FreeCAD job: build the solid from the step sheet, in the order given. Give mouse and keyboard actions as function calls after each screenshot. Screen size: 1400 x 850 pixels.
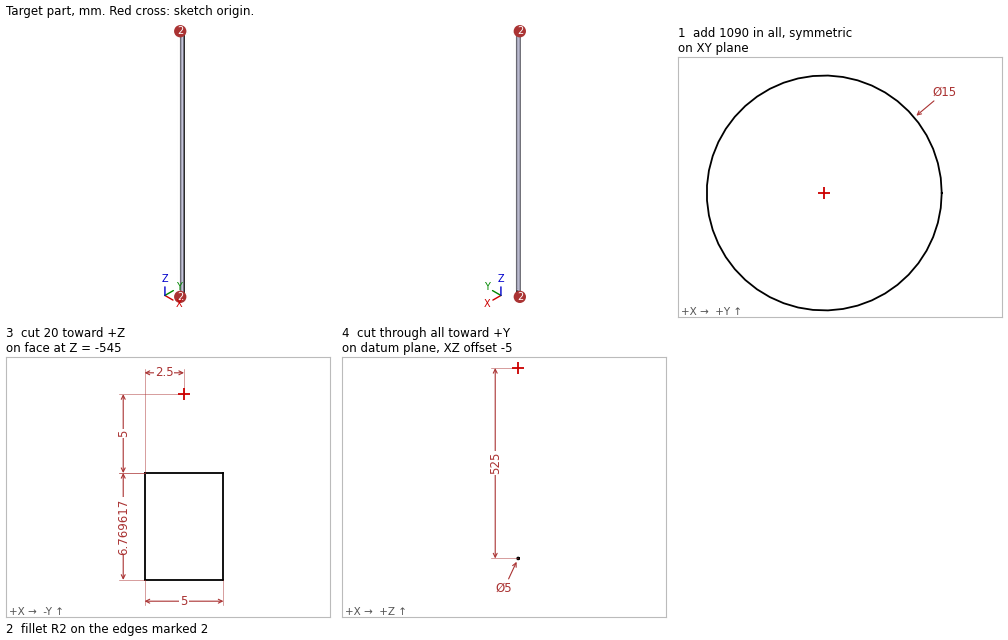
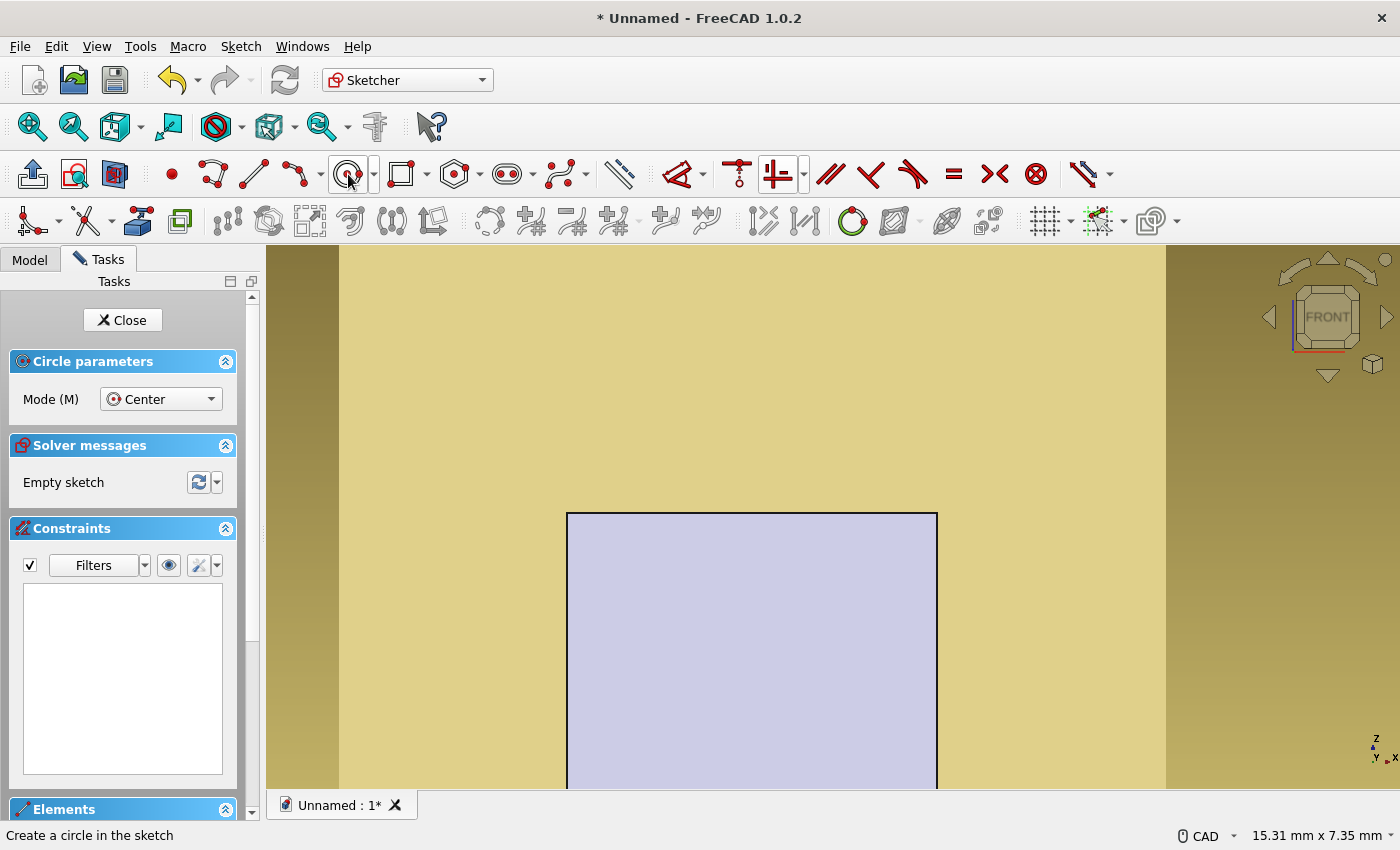
click(752, 513)
click(883, 382)
key(Escape)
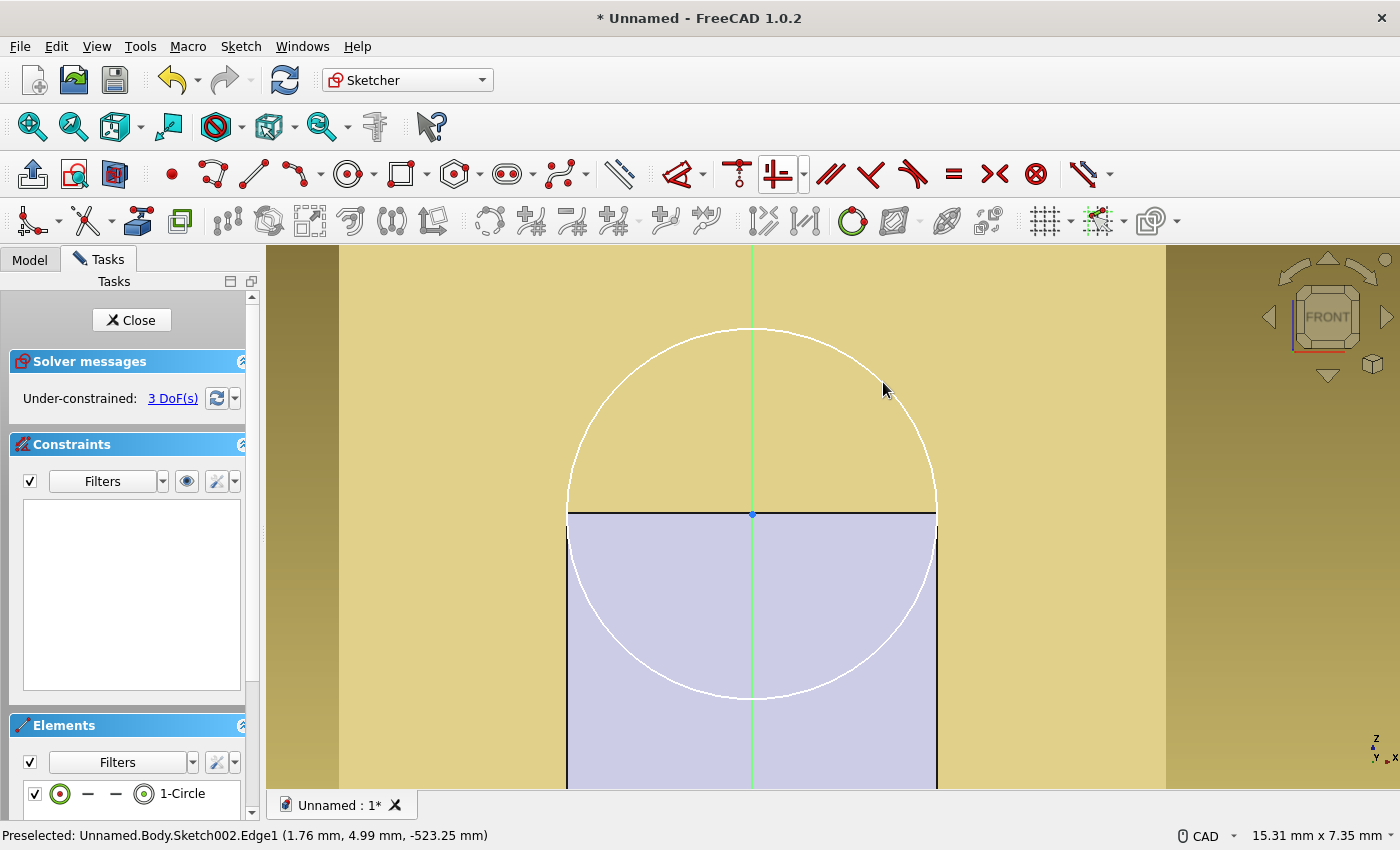
click(752, 514)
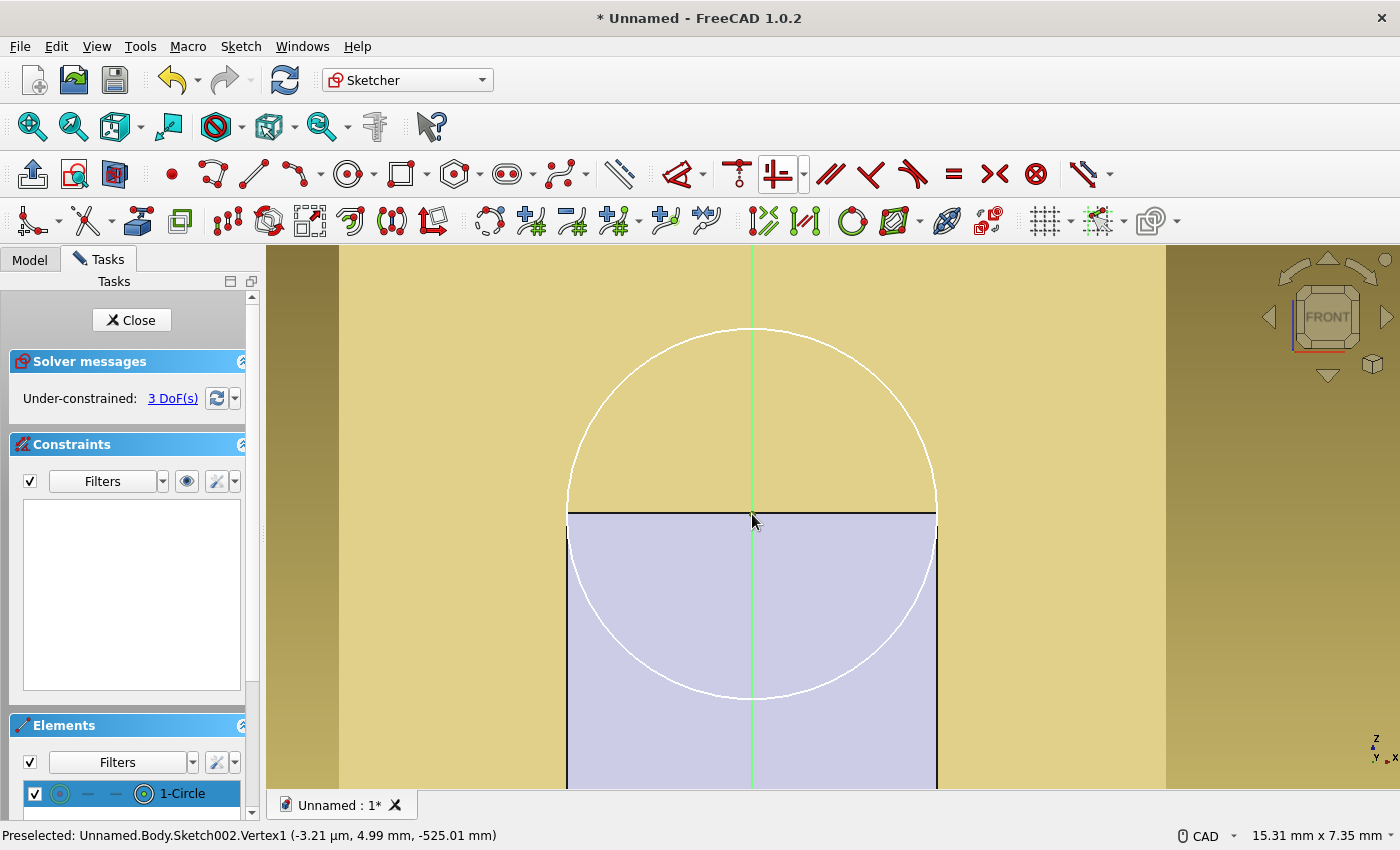
click(752, 656)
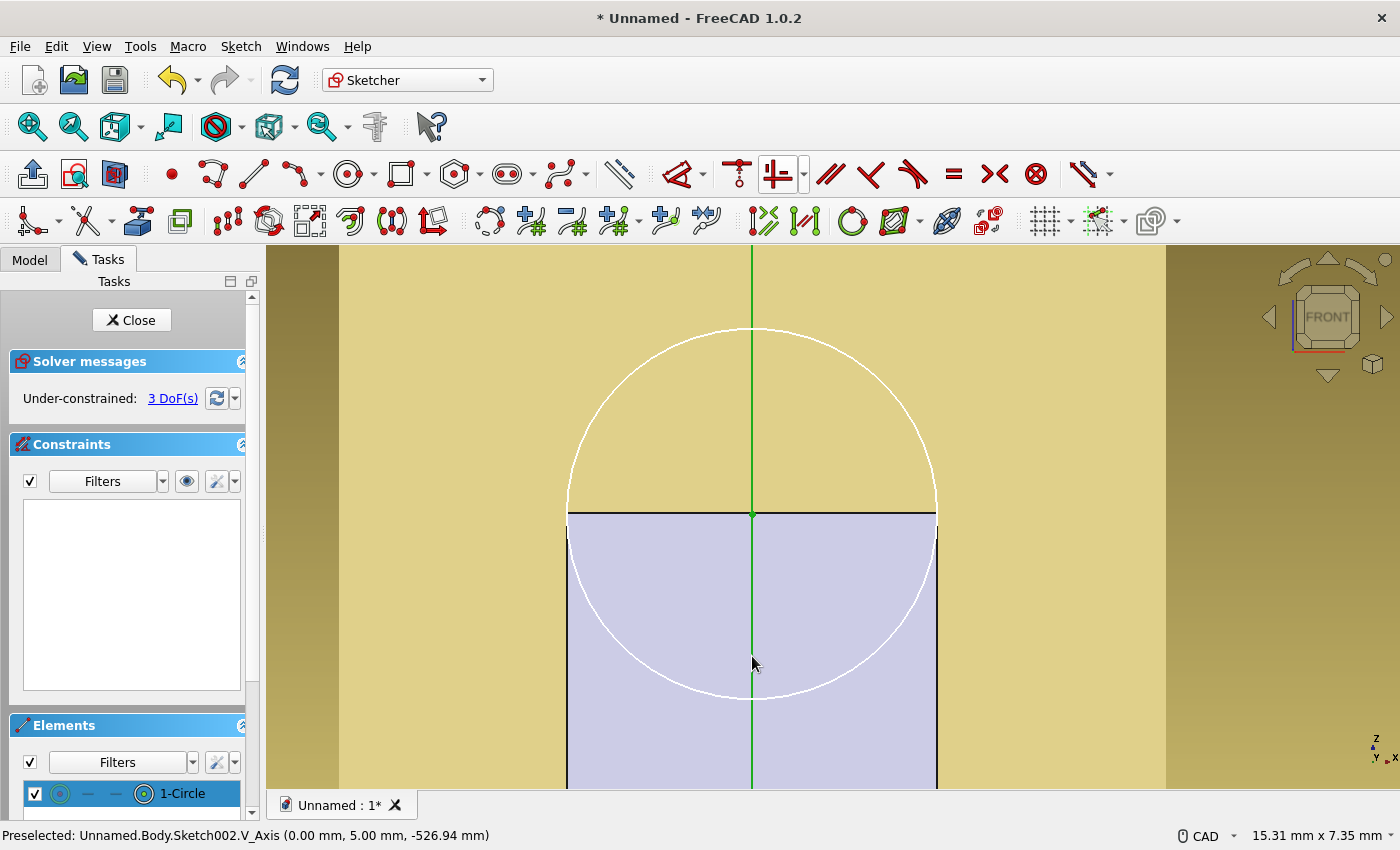
key(c)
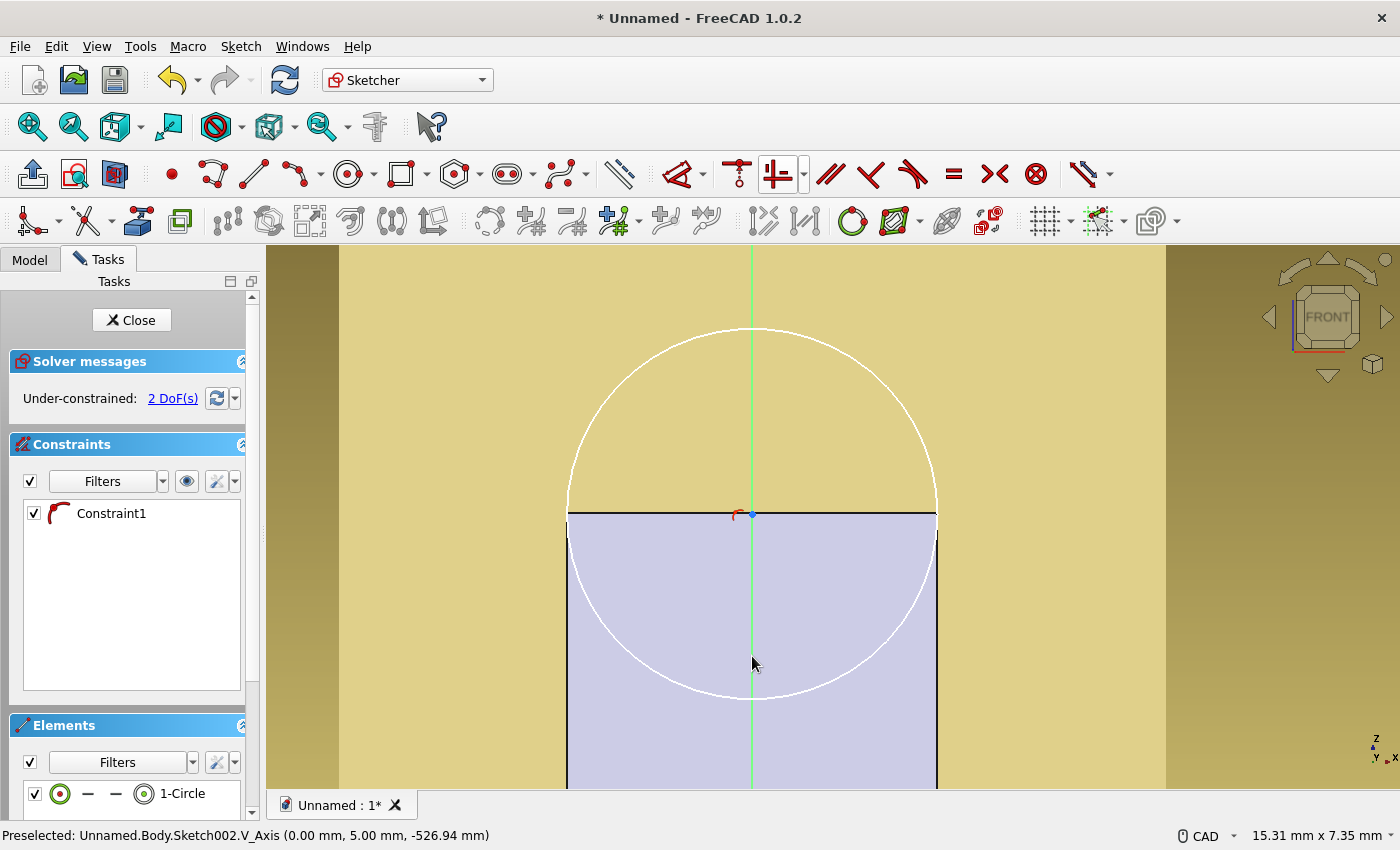
click(676, 174)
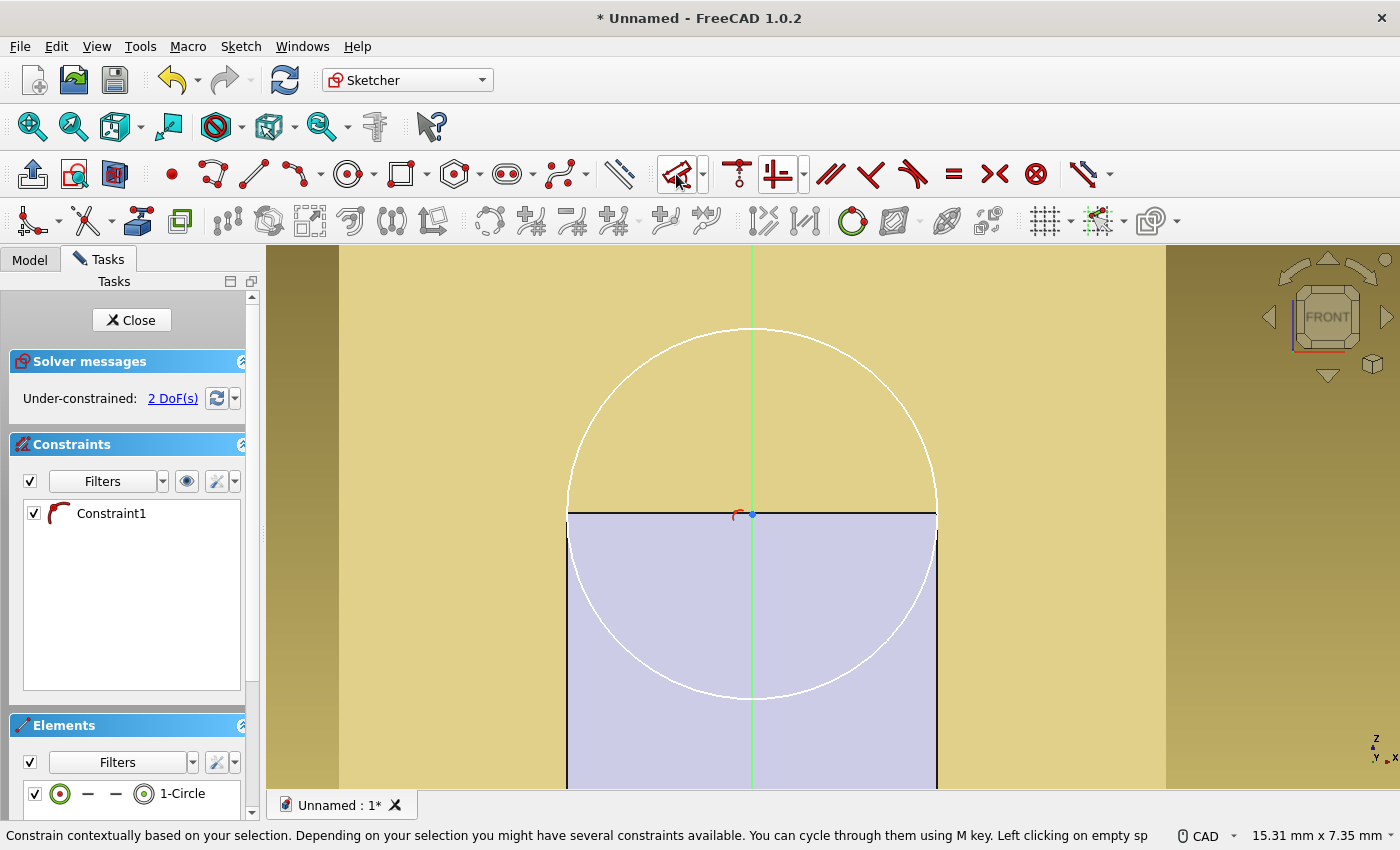
click(883, 383)
click(906, 360)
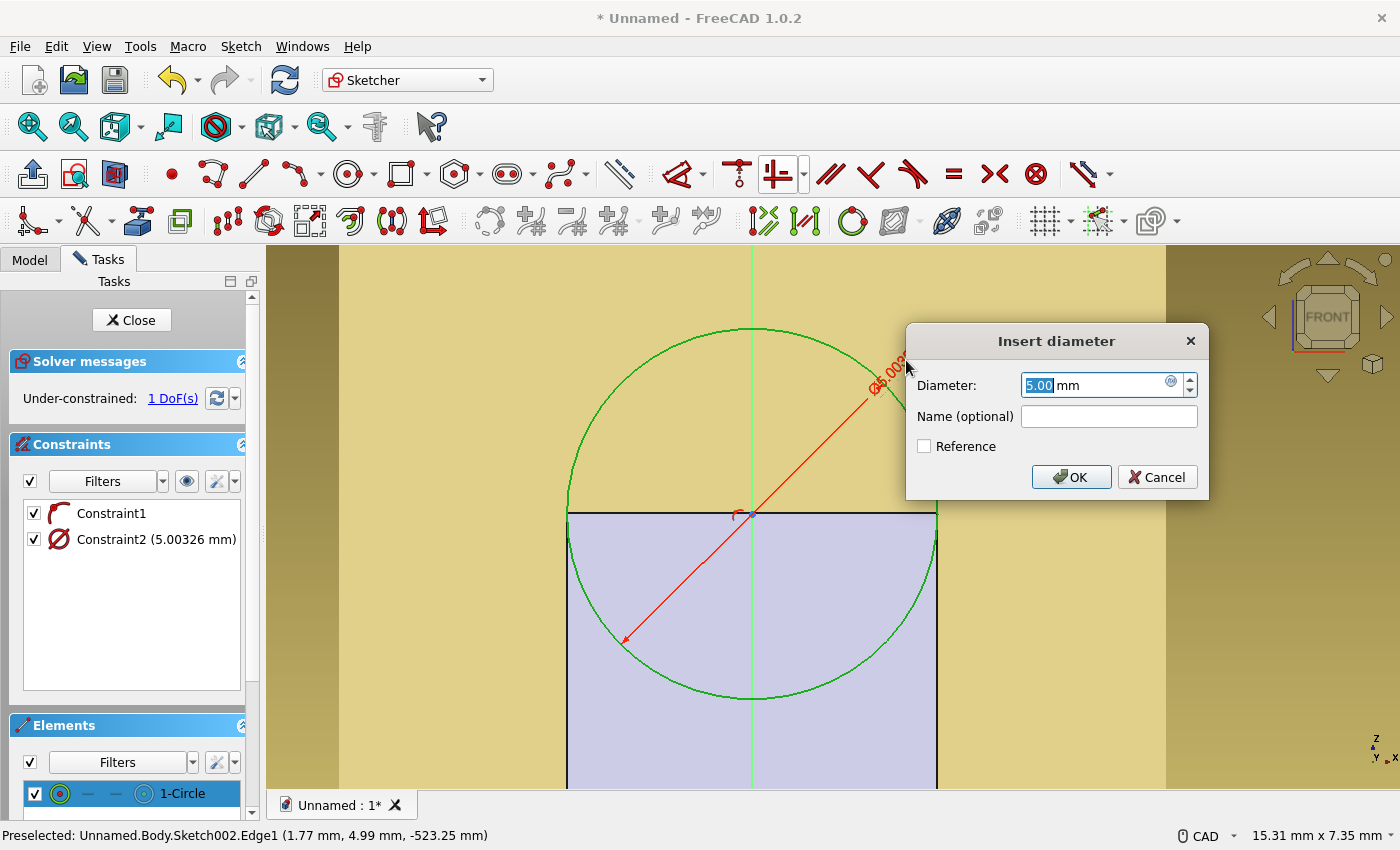
text(5)
key(Return)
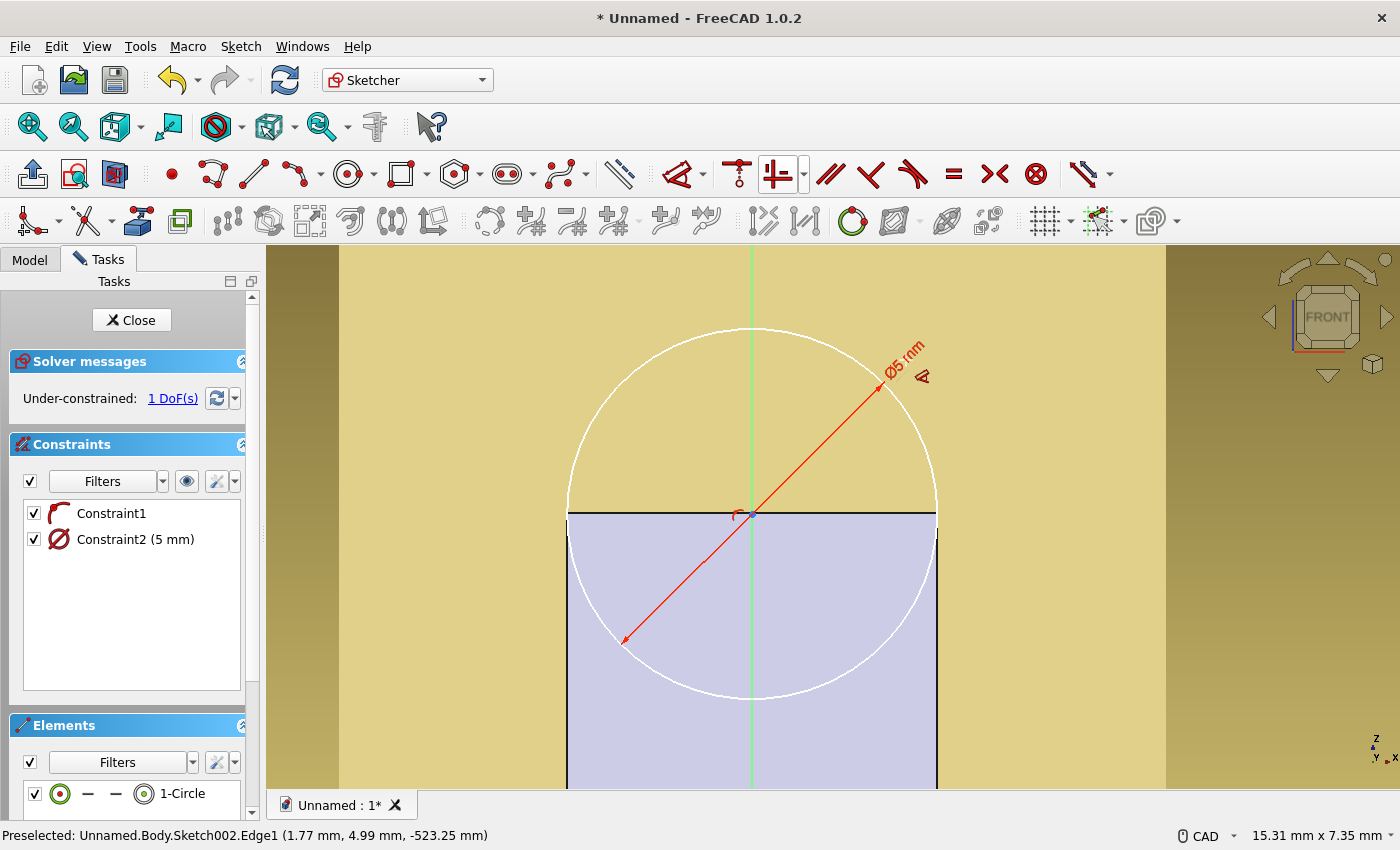
click(752, 514)
click(786, 393)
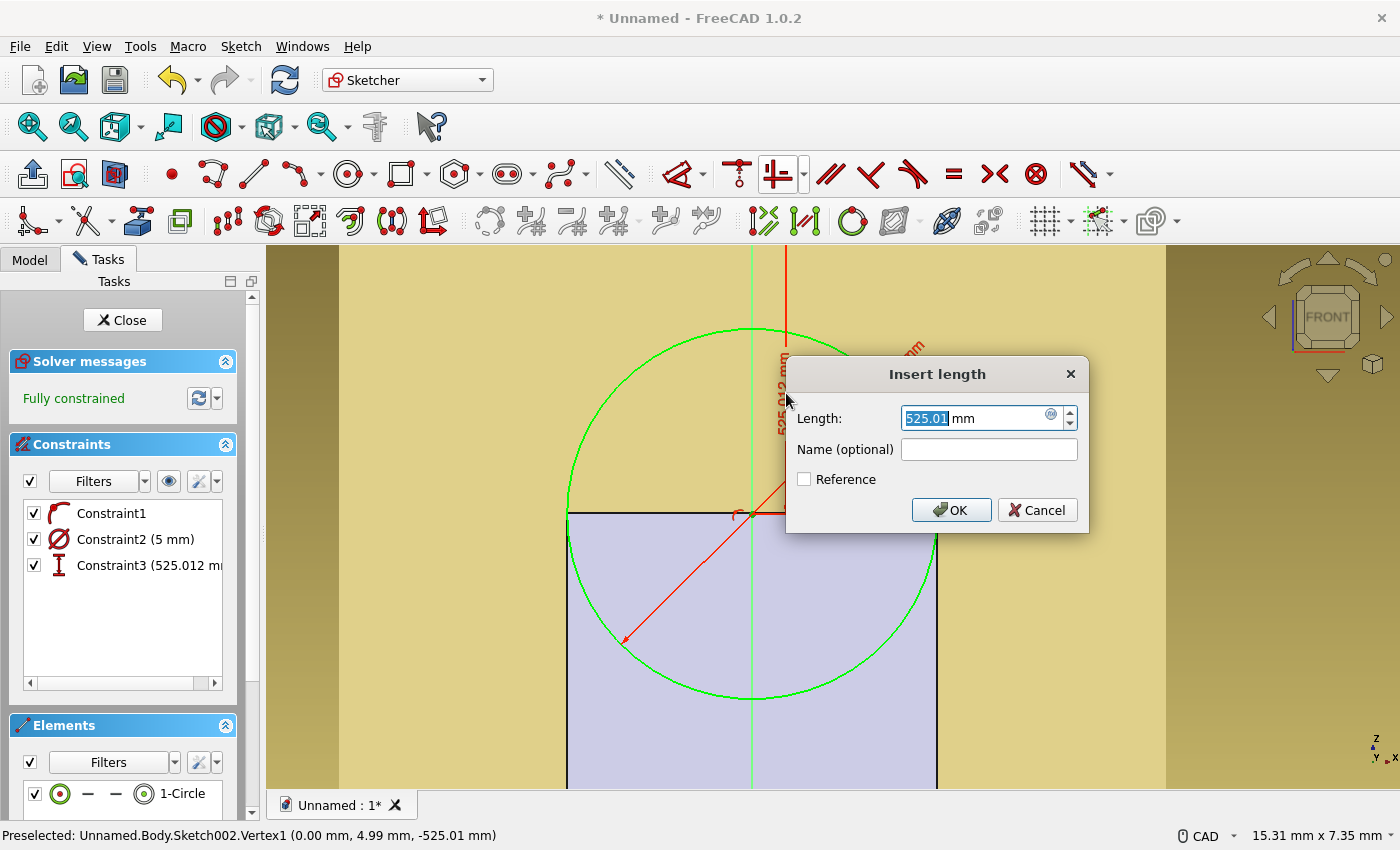
text(525)
key(Return)
key(Escape)